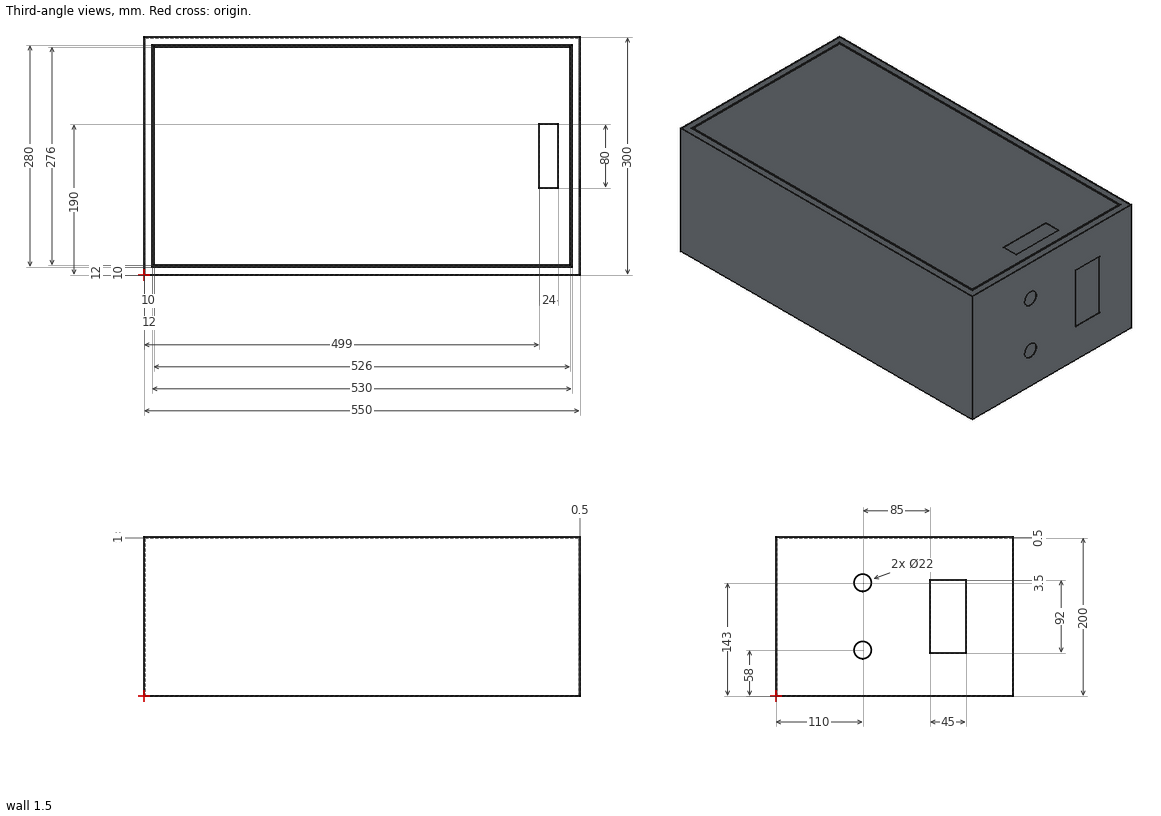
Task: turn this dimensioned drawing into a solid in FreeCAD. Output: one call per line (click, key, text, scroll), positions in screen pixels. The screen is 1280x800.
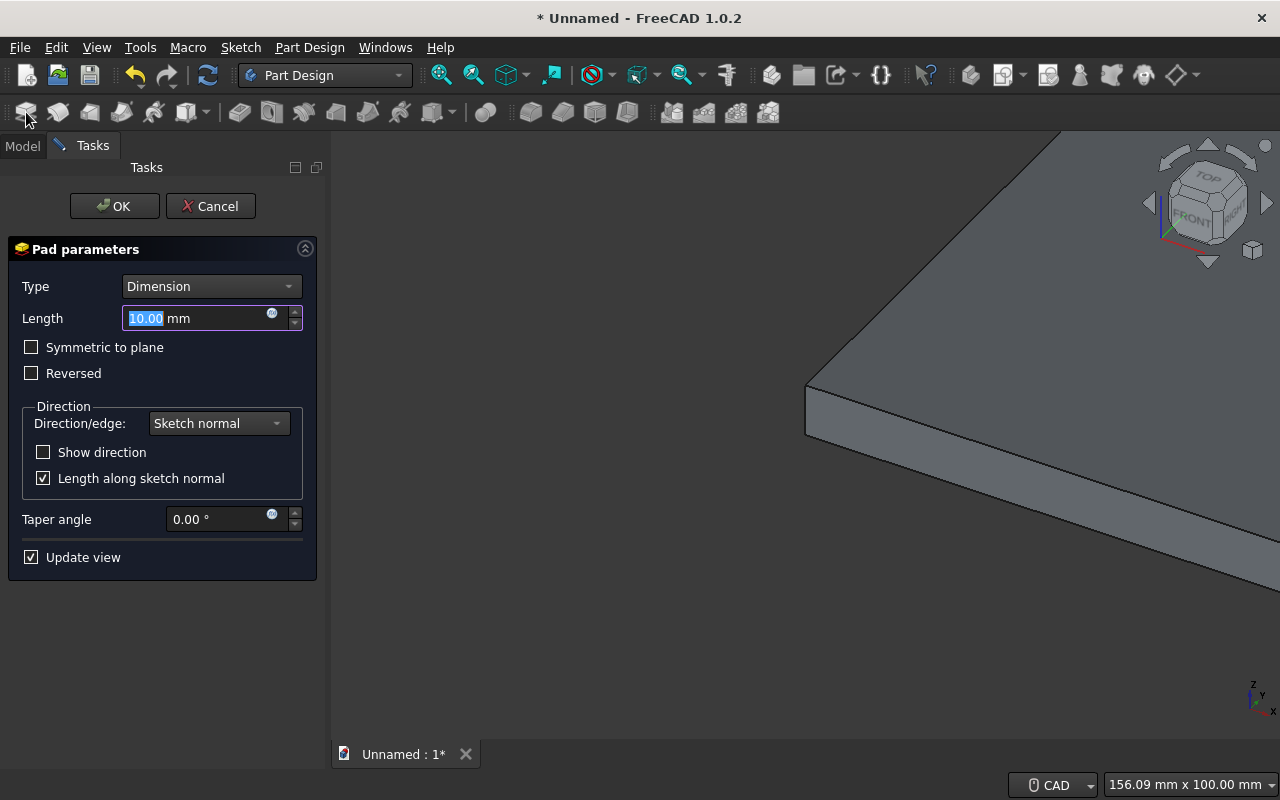
text(200)
key(Tab)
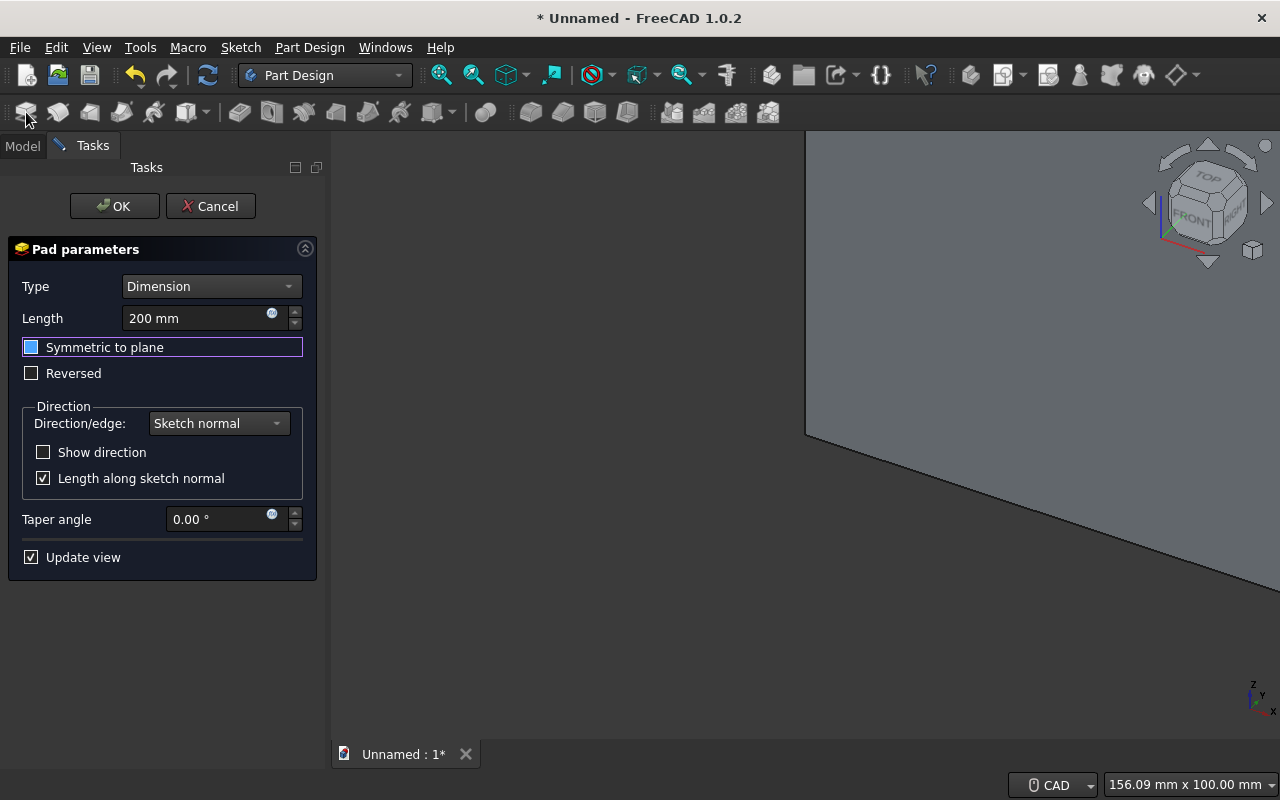
click(115, 206)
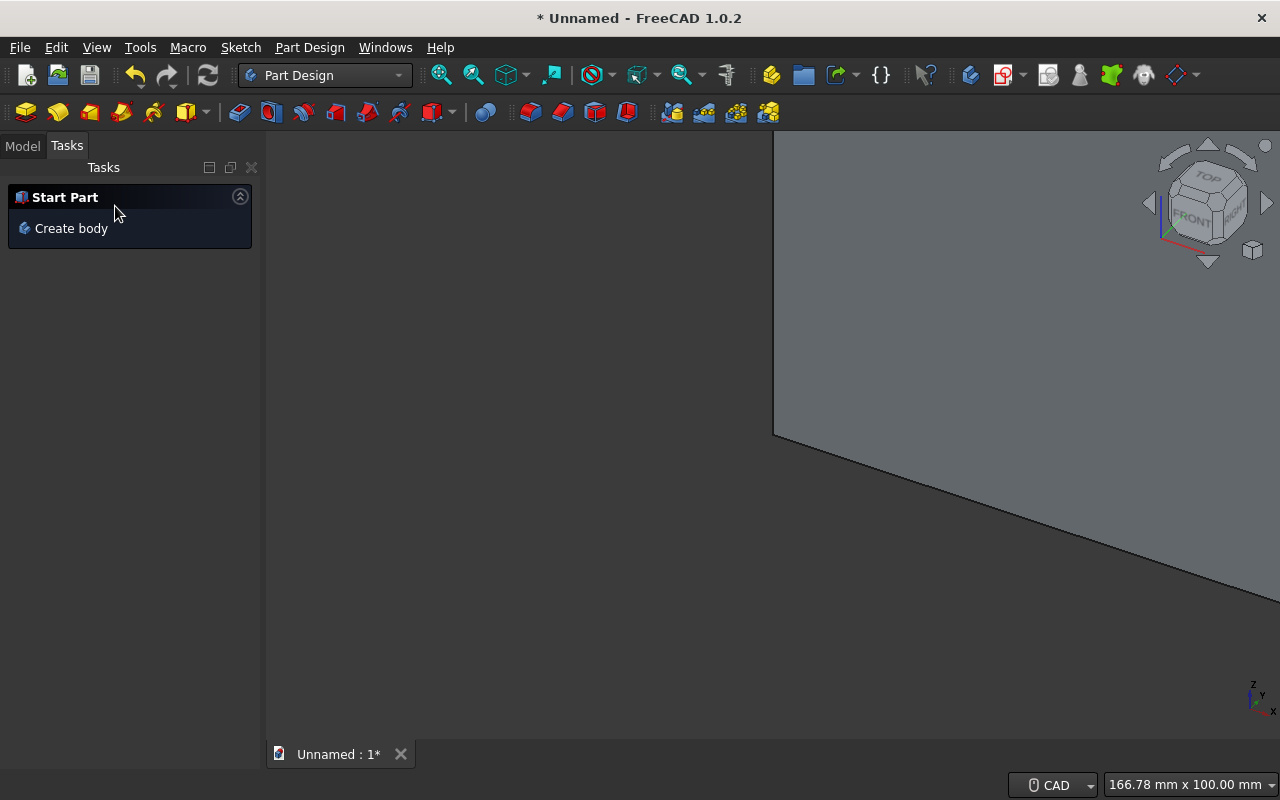
click(442, 76)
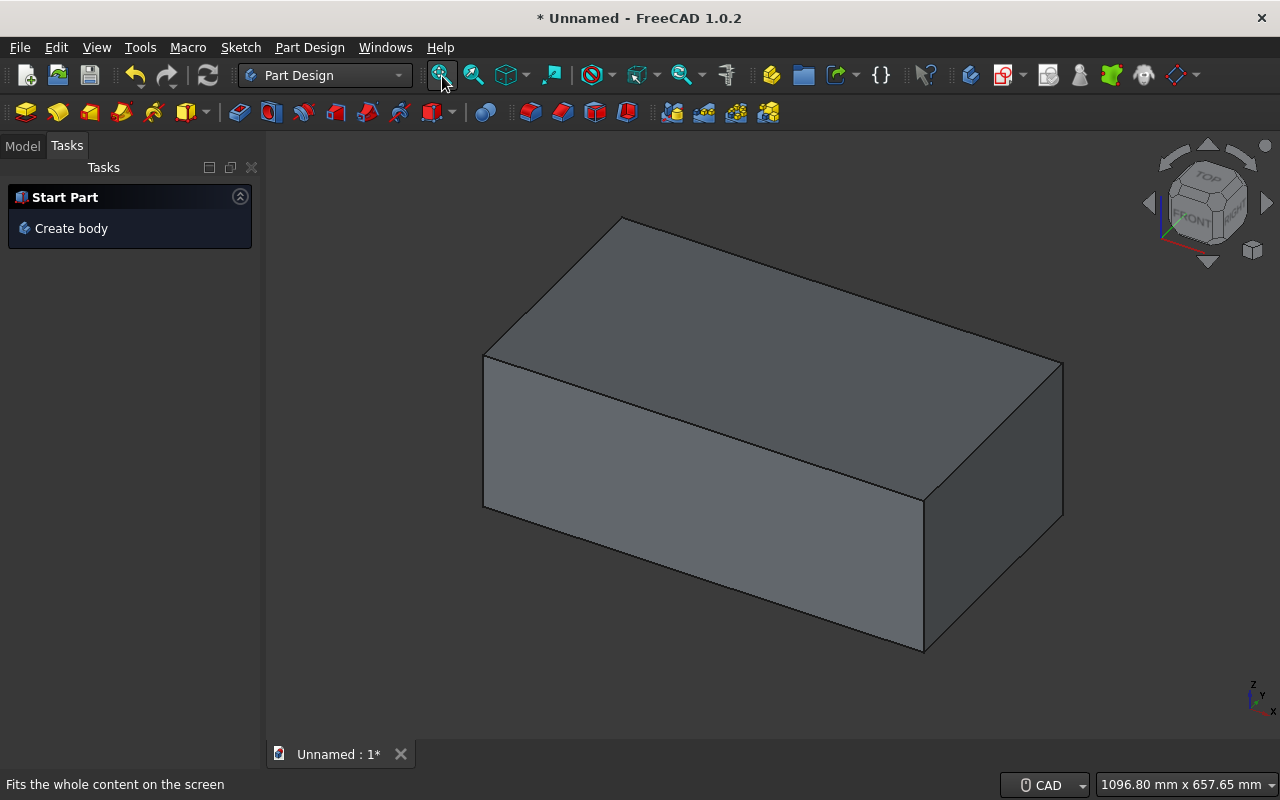
click(836, 379)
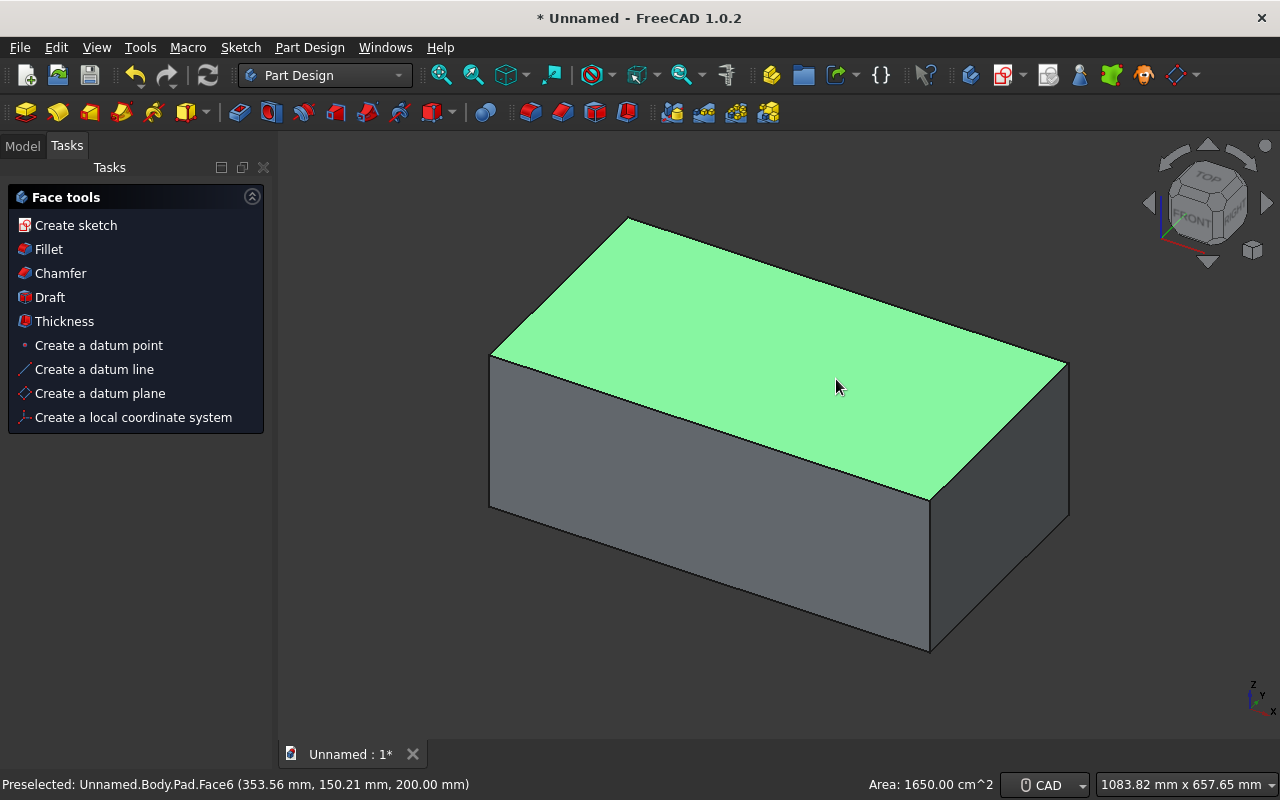
click(628, 112)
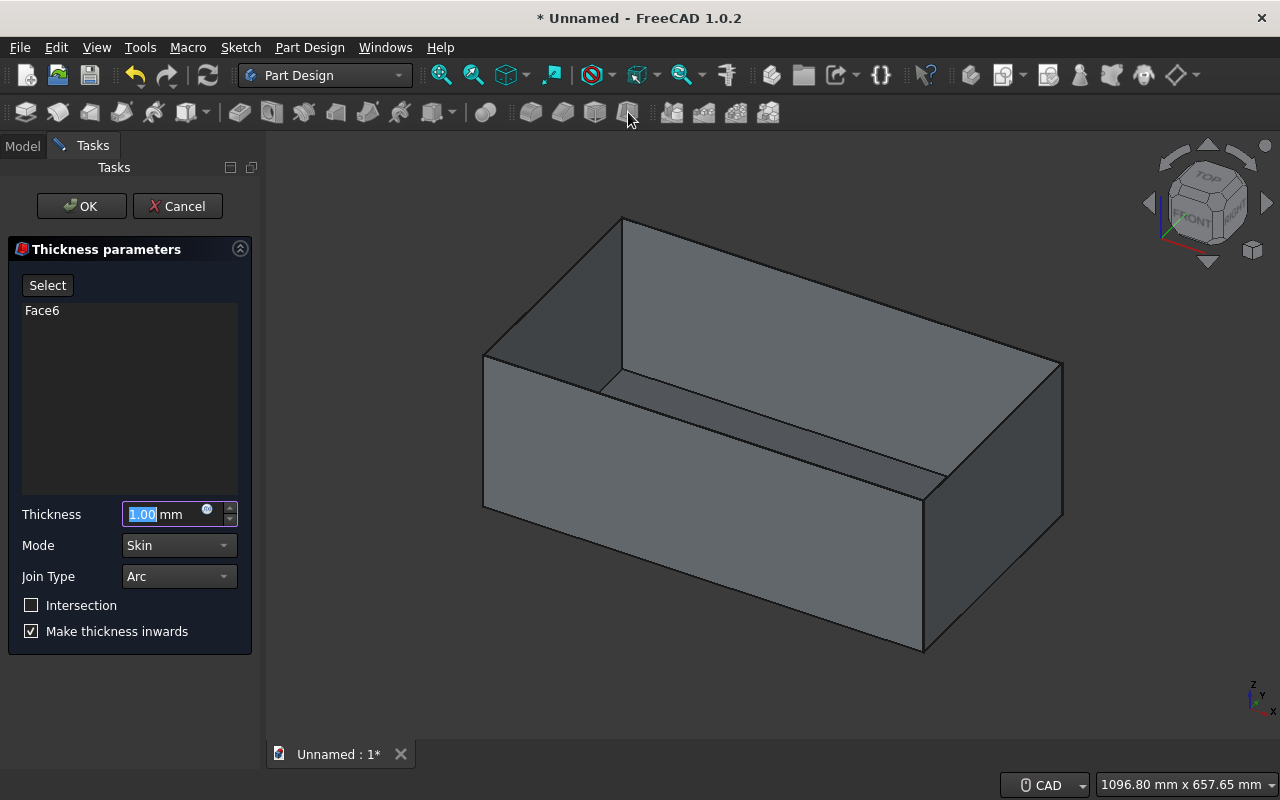
text(1.5)
key(Tab)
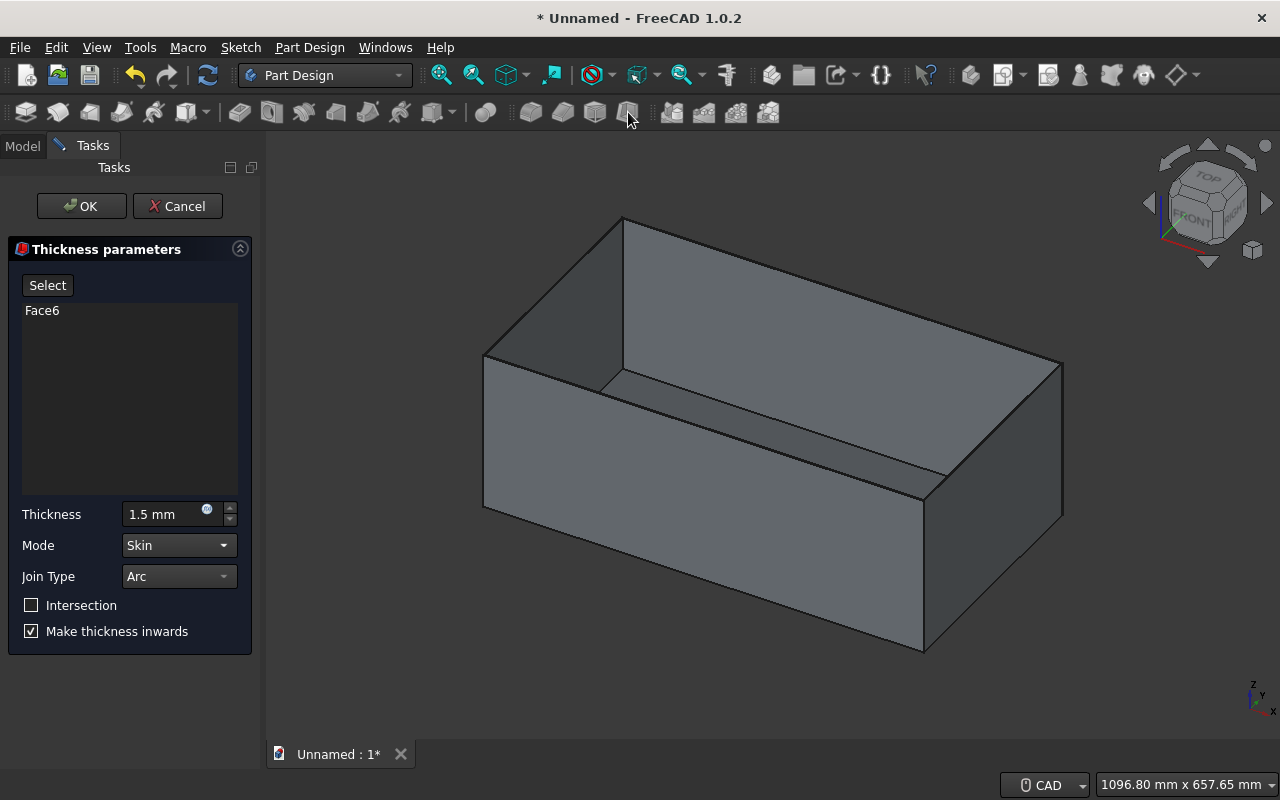
click(180, 576)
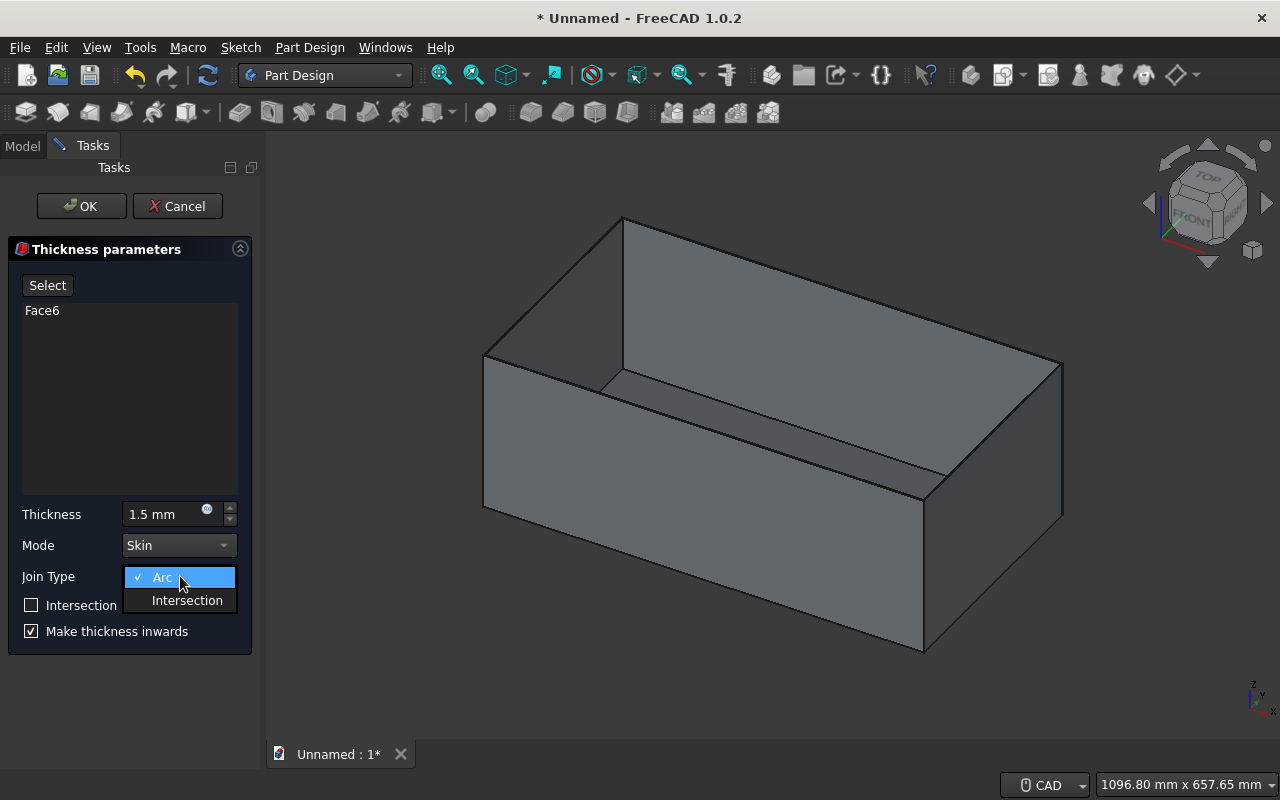
click(179, 600)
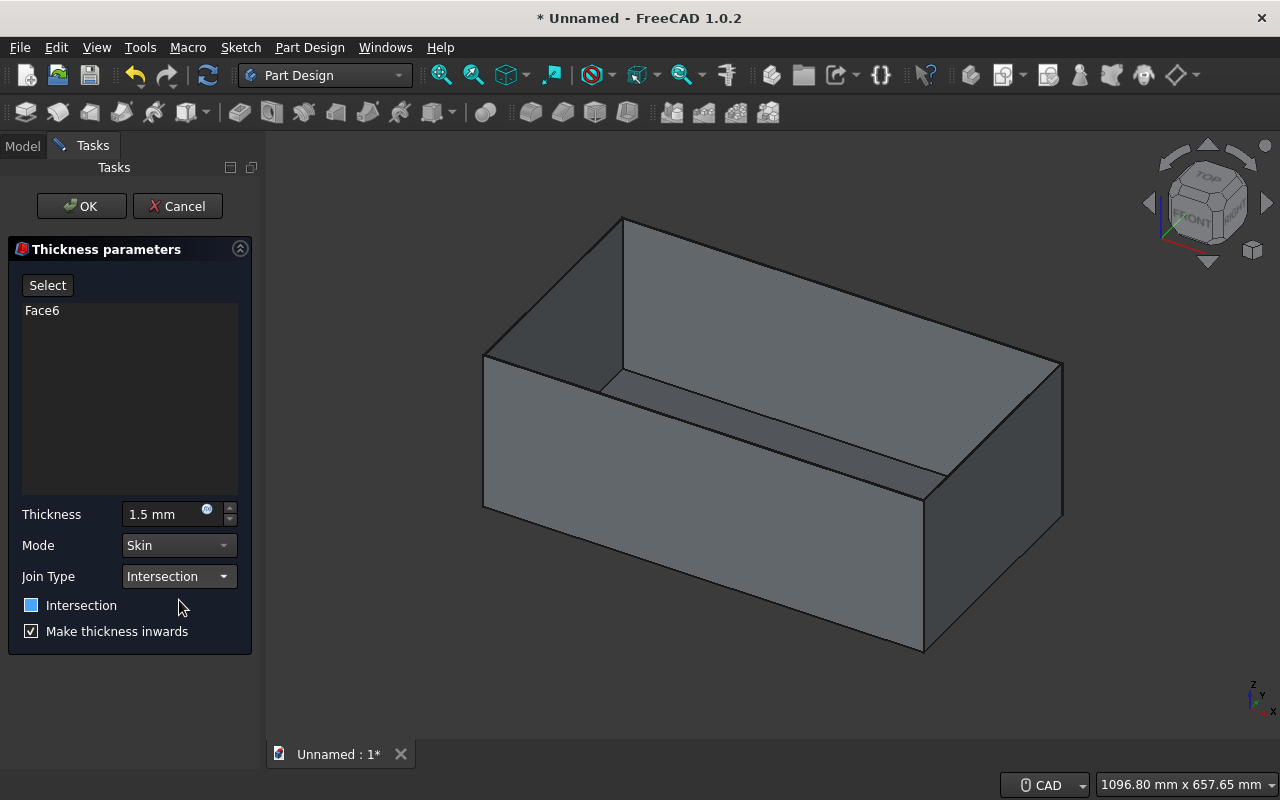
click(82, 206)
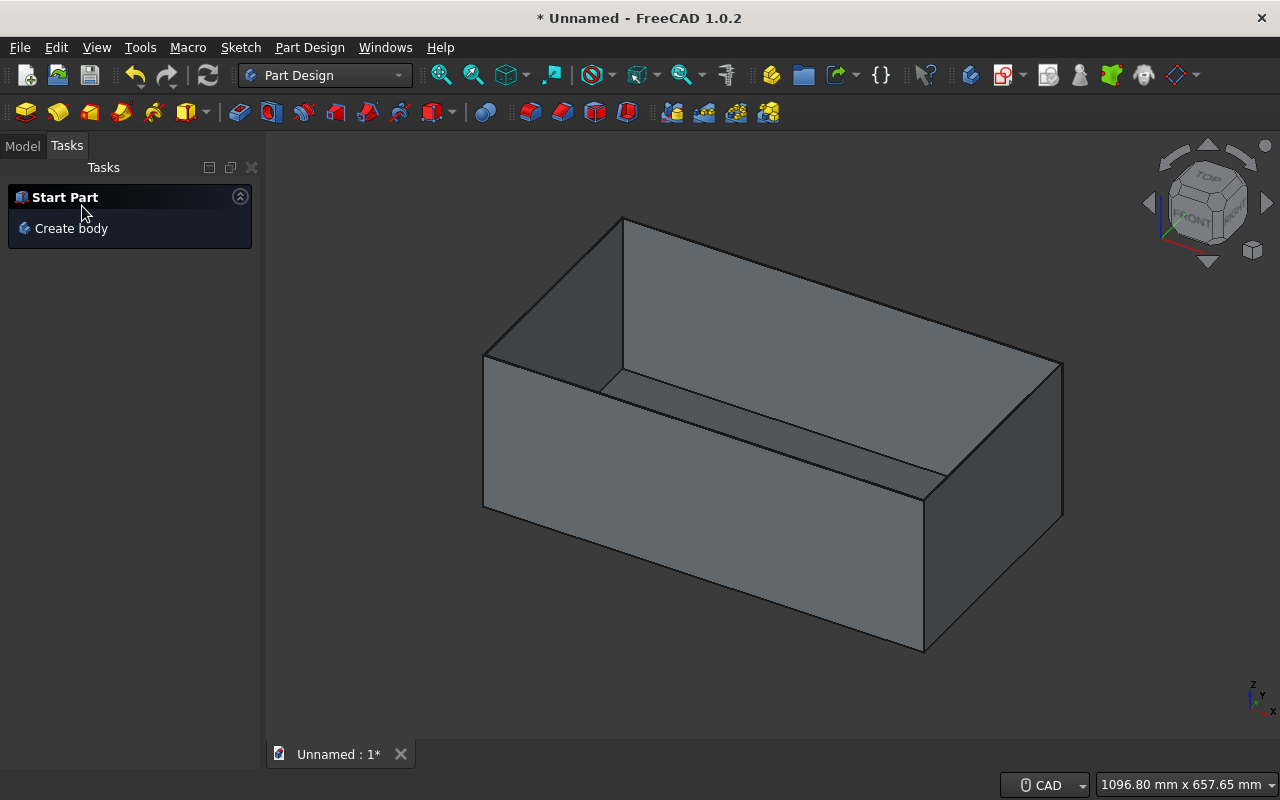
scroll(970, 454, up, 15)